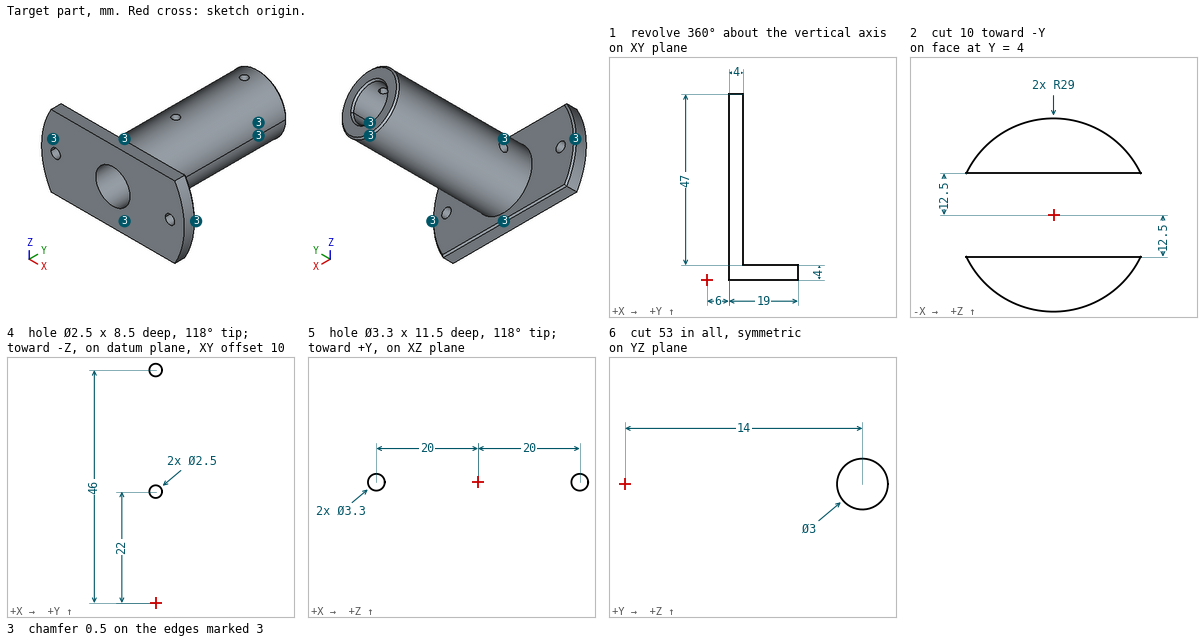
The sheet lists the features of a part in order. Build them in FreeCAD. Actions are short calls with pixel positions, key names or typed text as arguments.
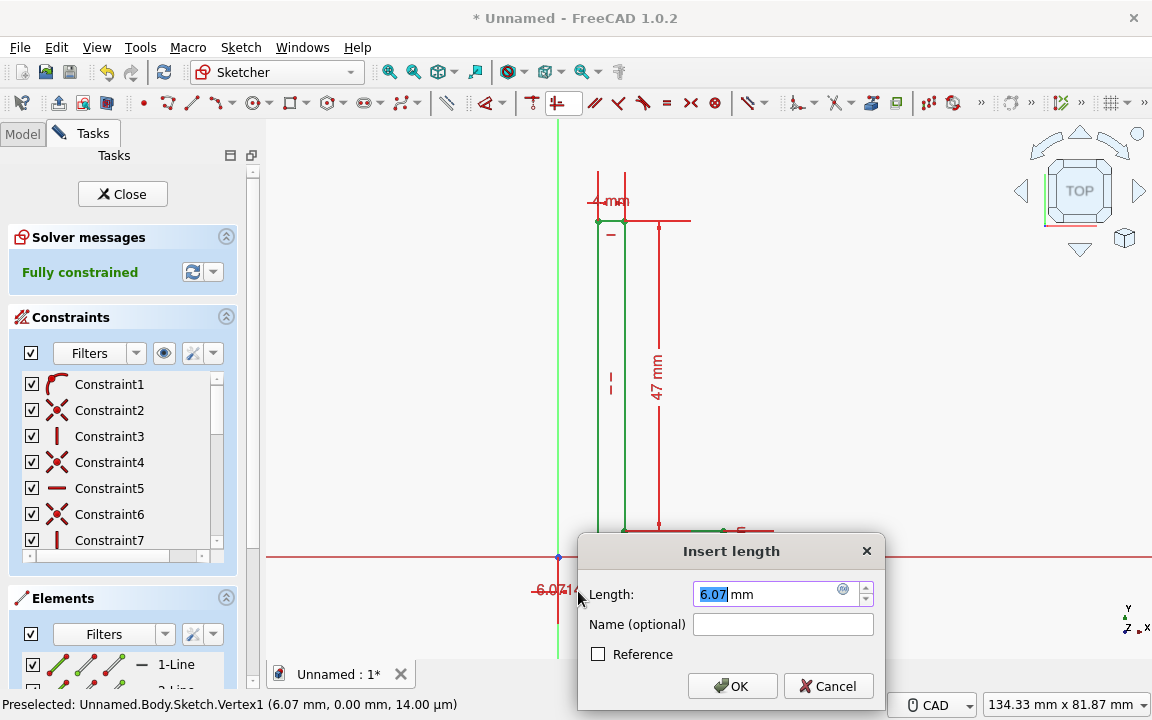
text(6)
key(Return)
key(Escape)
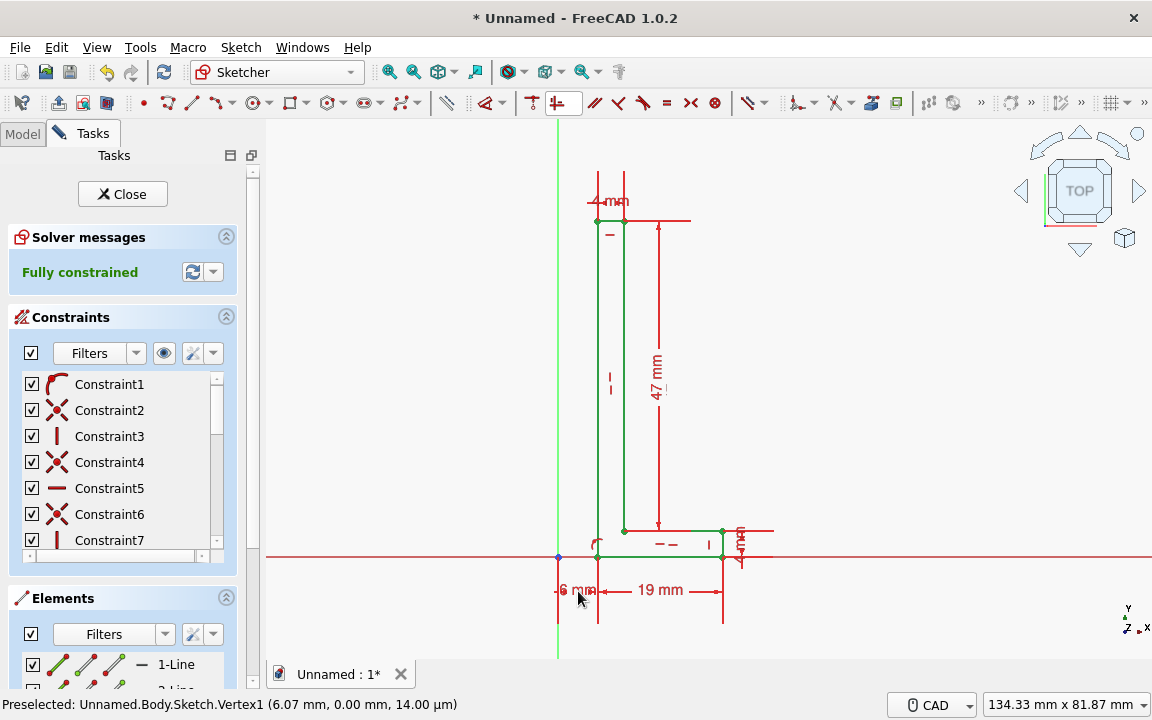
click(123, 194)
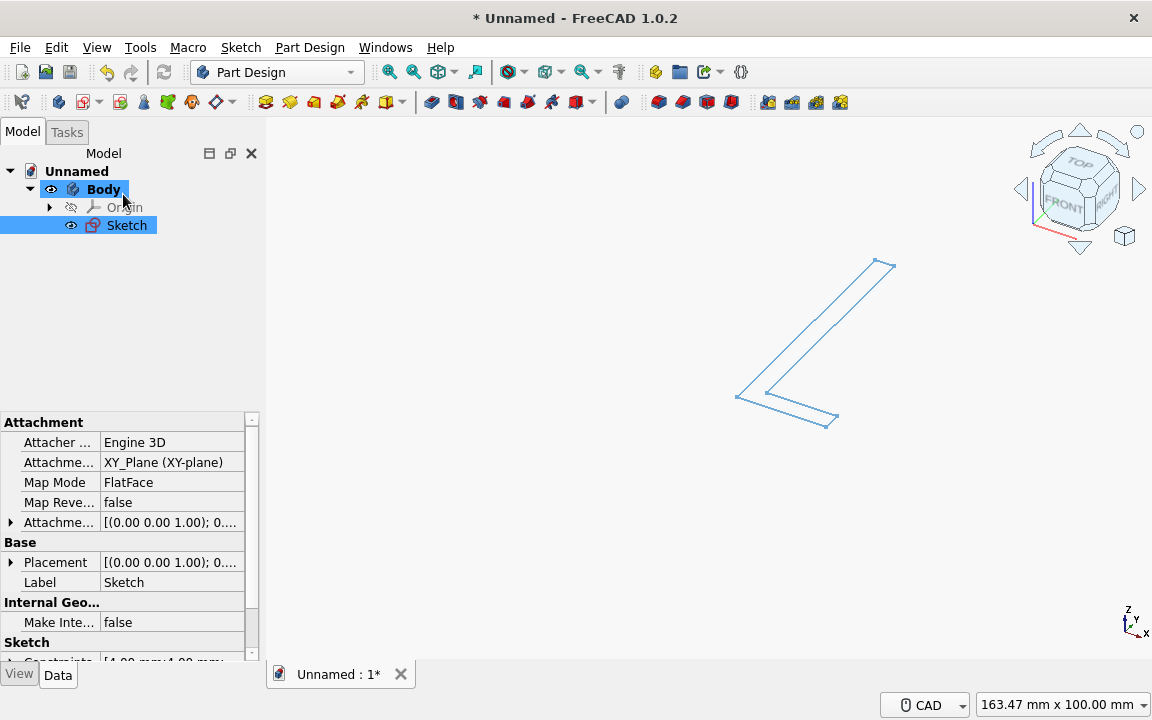
click(290, 102)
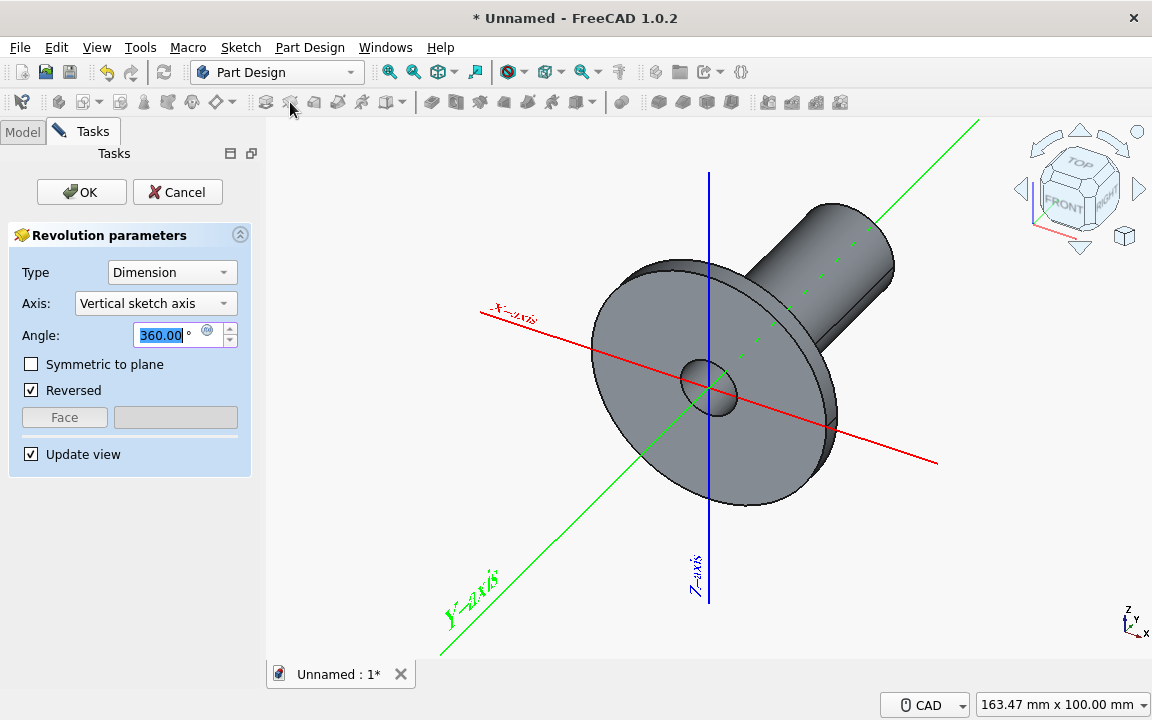
click(82, 192)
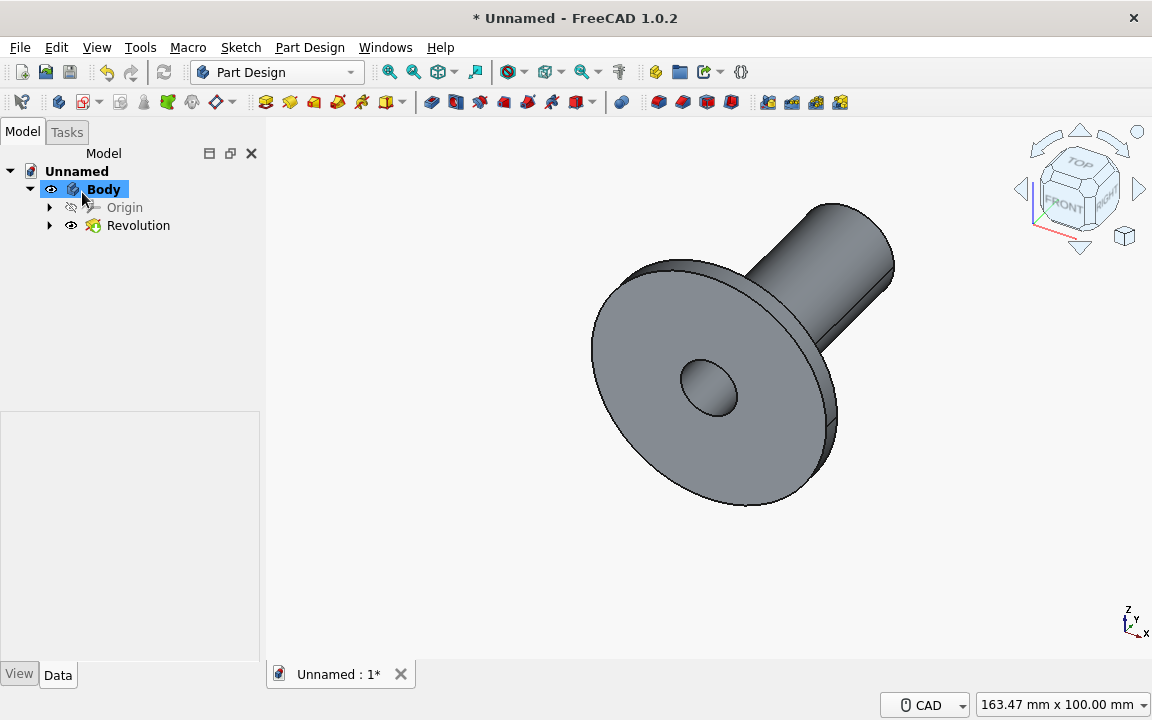
click(390, 72)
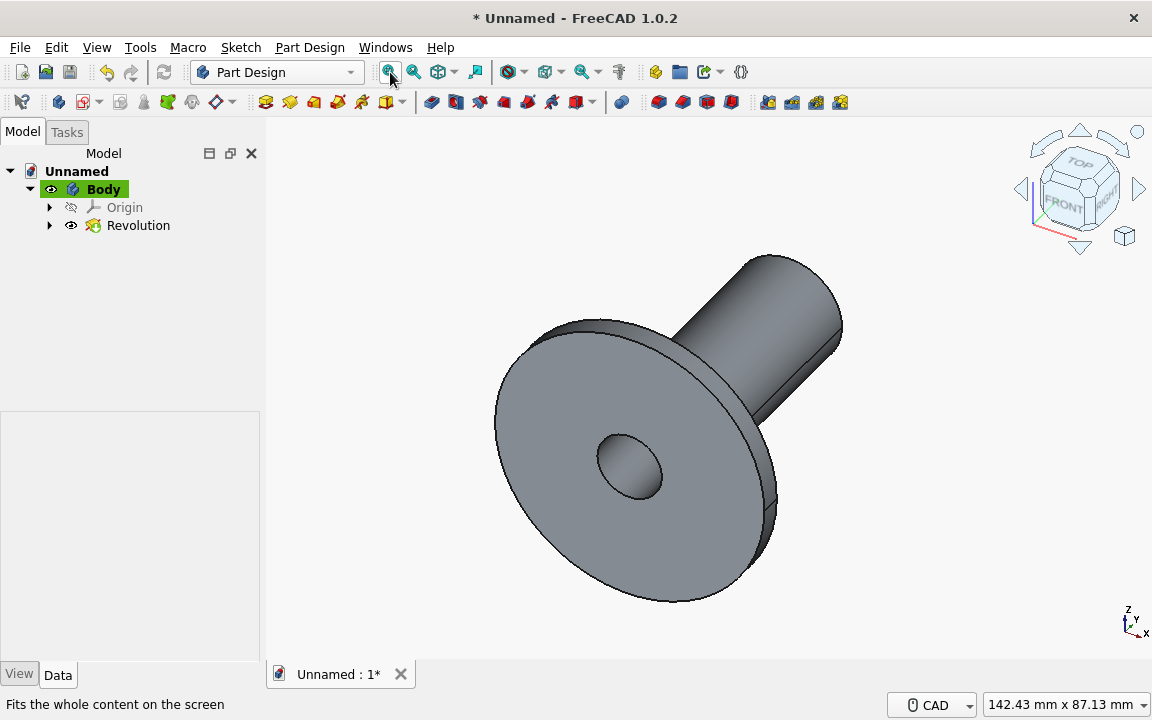
key(4)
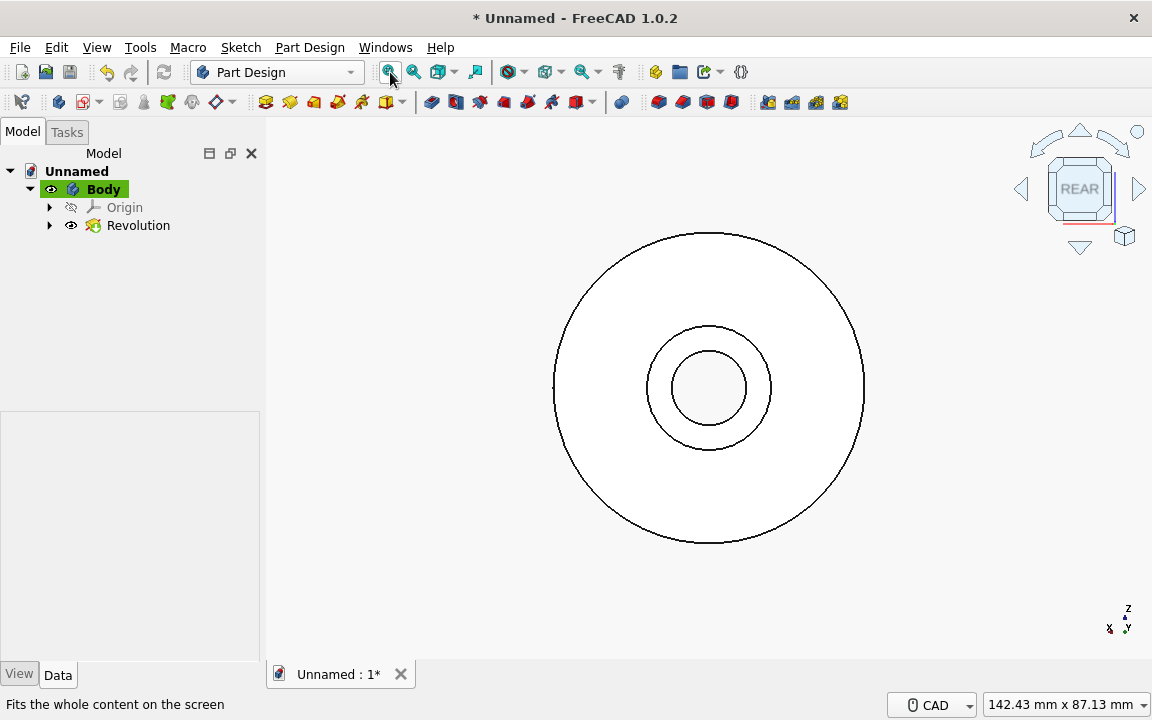
click(665, 476)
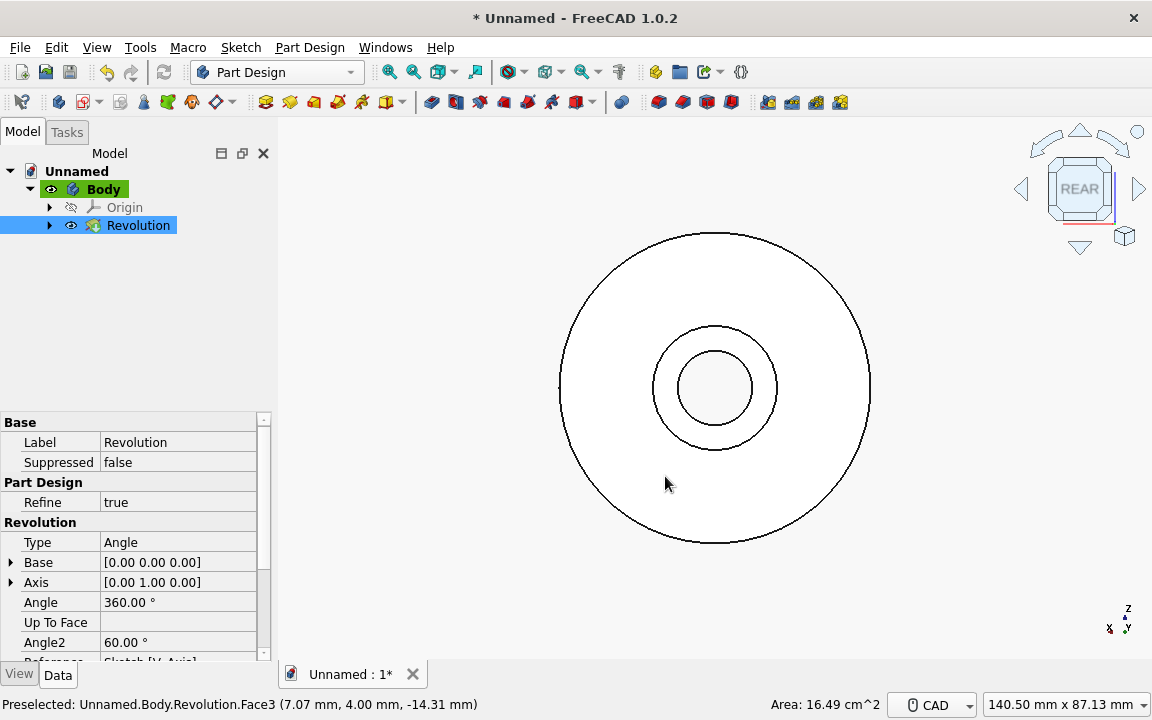
click(84, 102)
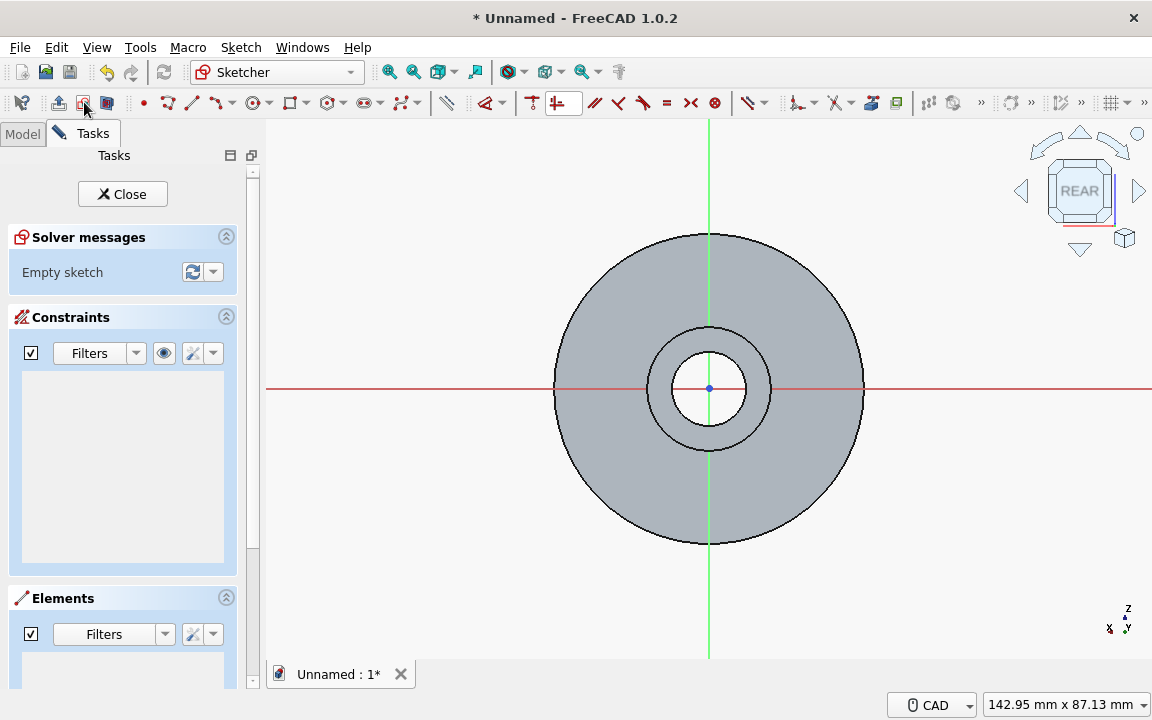
click(192, 104)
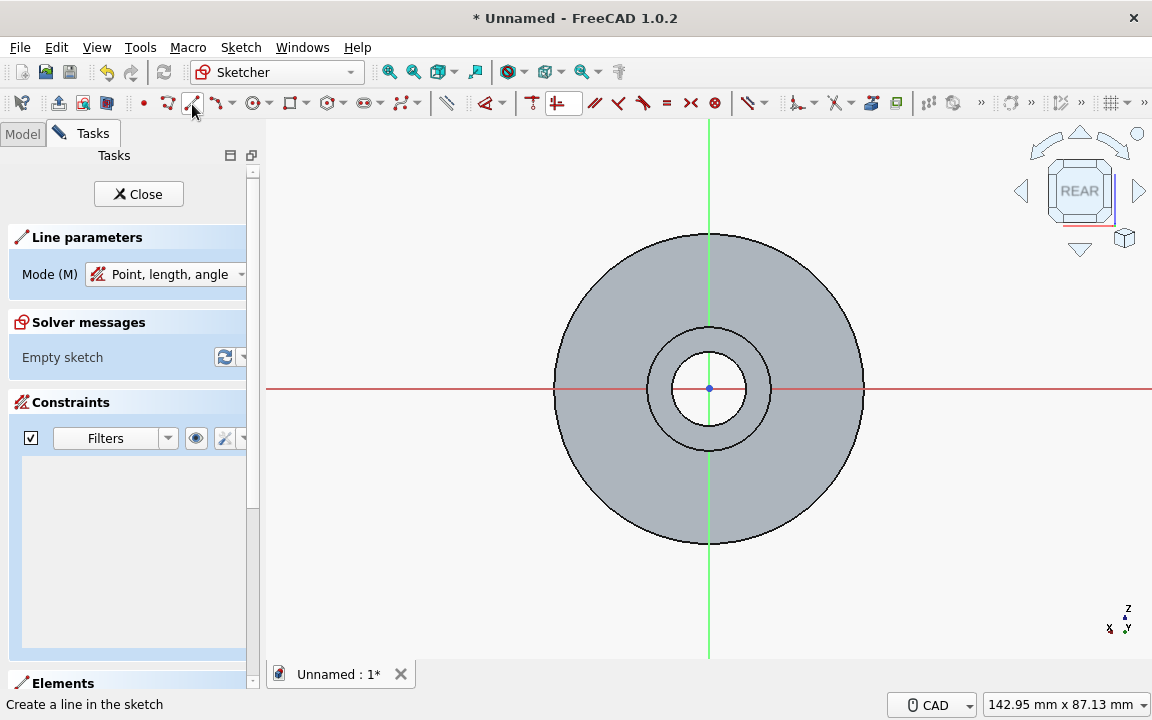
click(547, 312)
click(871, 312)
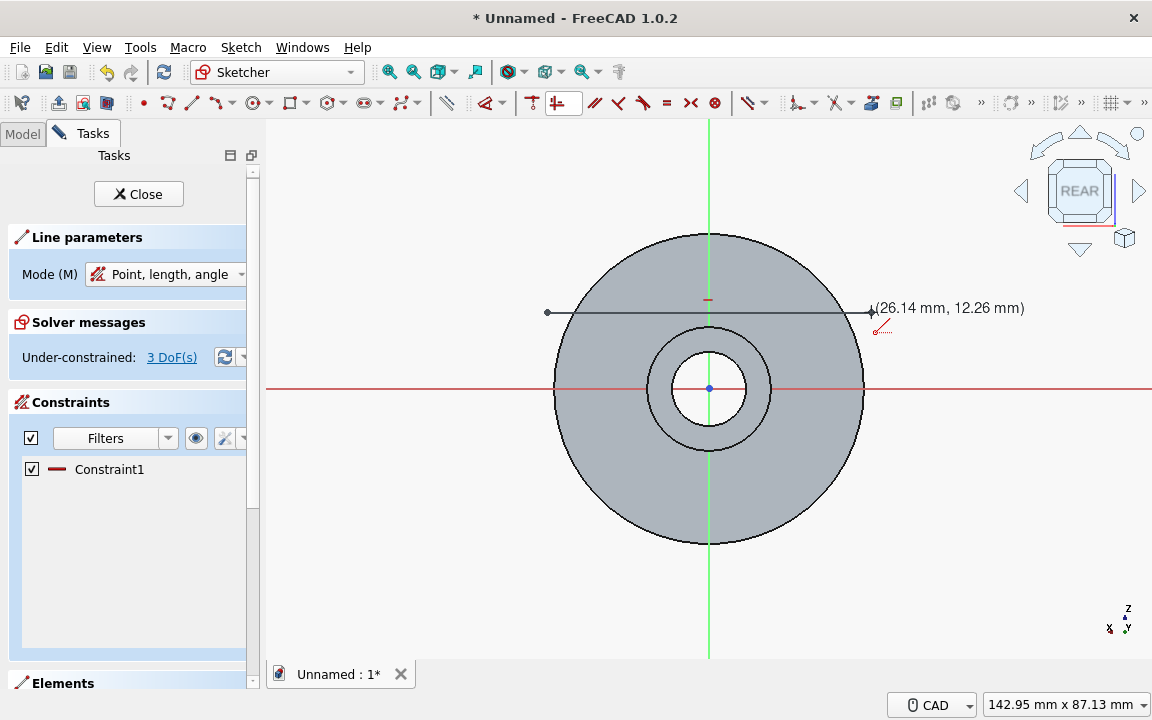
click(216, 104)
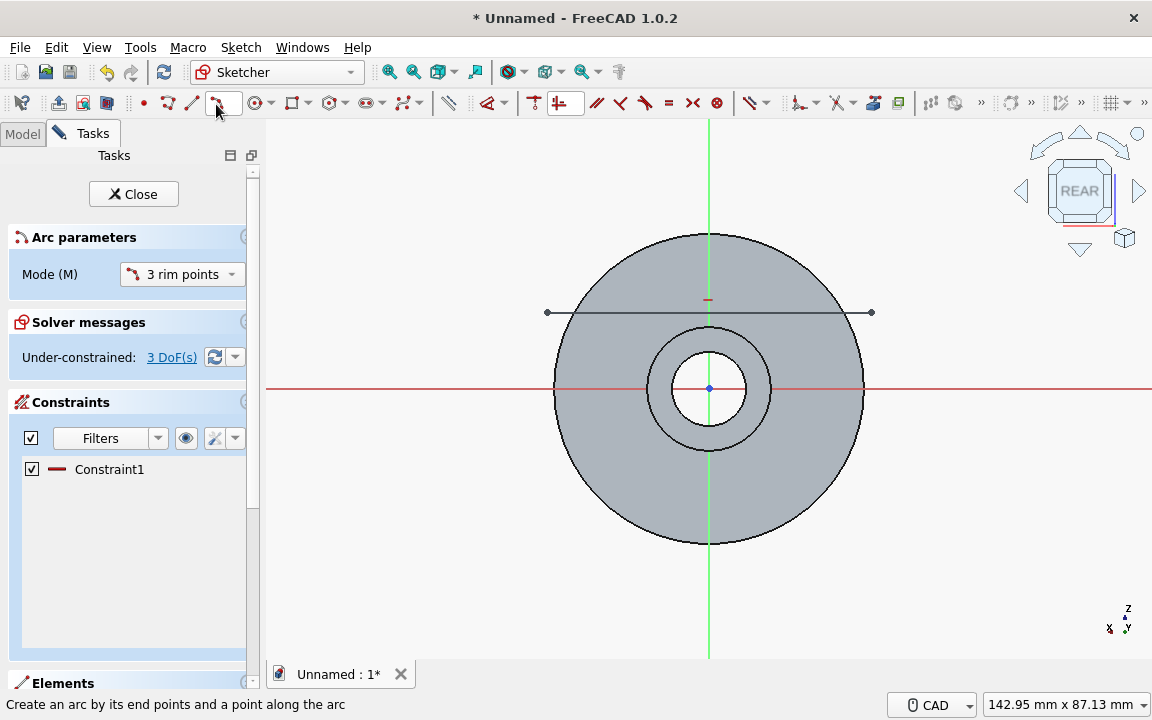
click(871, 313)
click(547, 313)
click(749, 214)